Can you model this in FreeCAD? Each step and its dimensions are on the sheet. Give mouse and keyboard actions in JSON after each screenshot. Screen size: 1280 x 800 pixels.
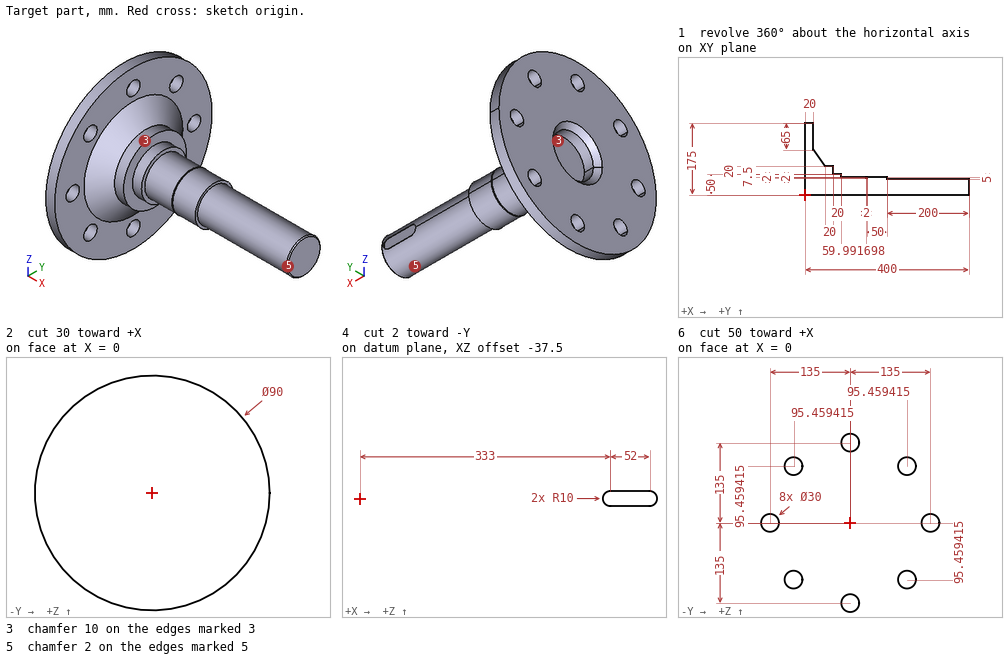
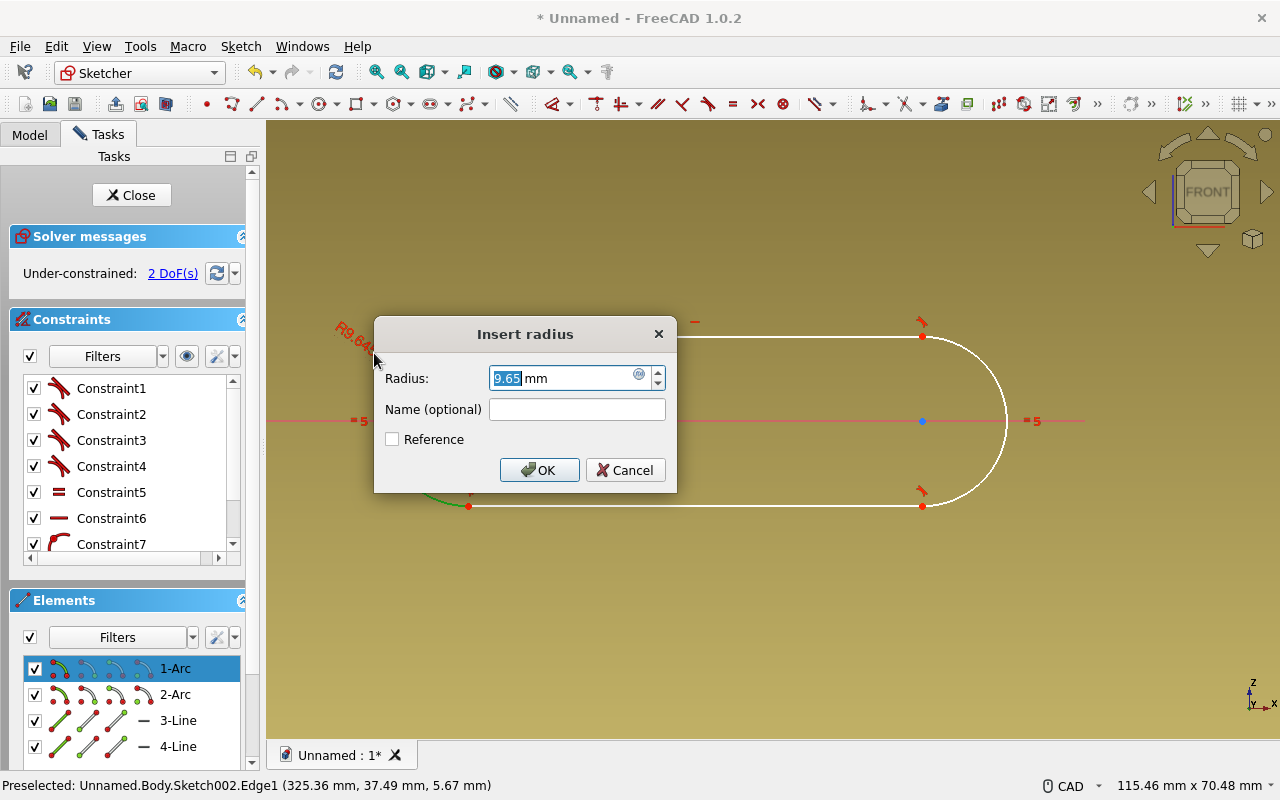
{"action": "type", "text": "10"}
{"action": "key", "text": "Return"}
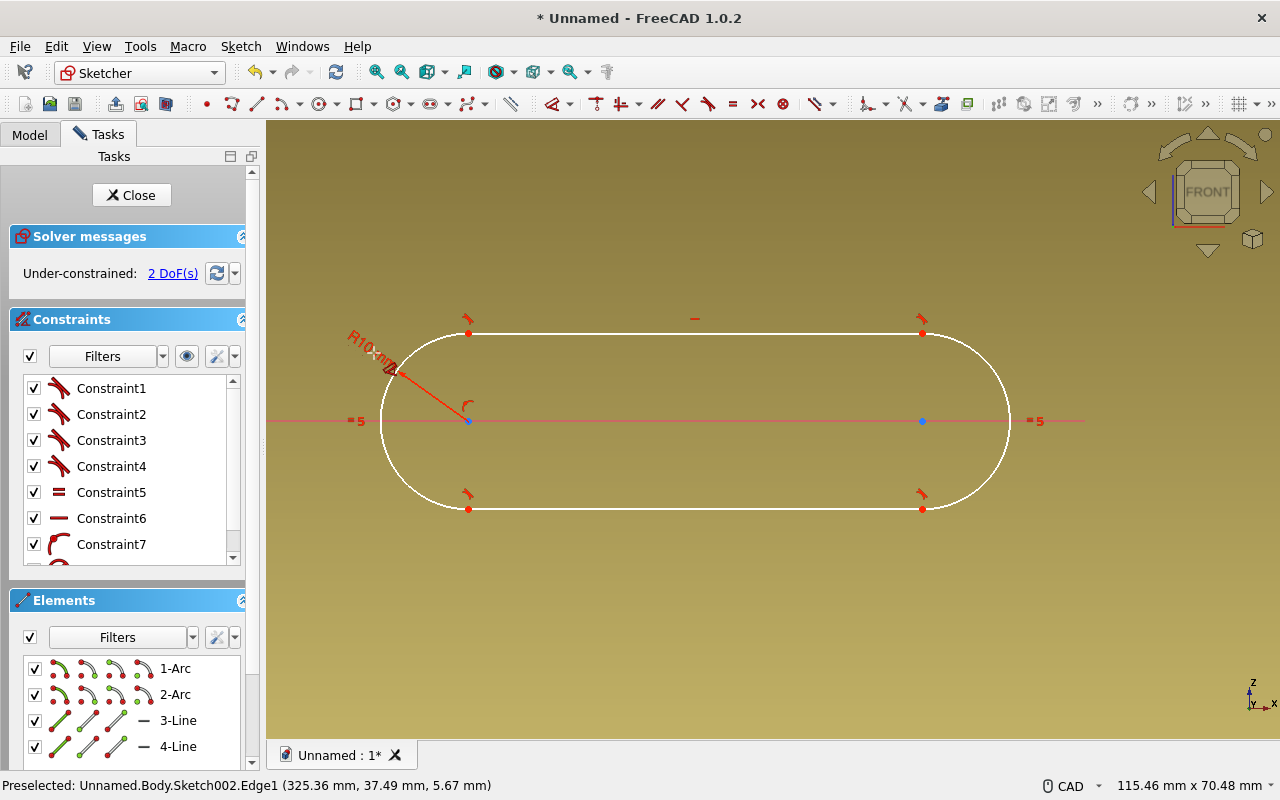
{"action": "left_click", "coordinate": [605, 334]}
{"action": "left_click", "coordinate": [695, 300]}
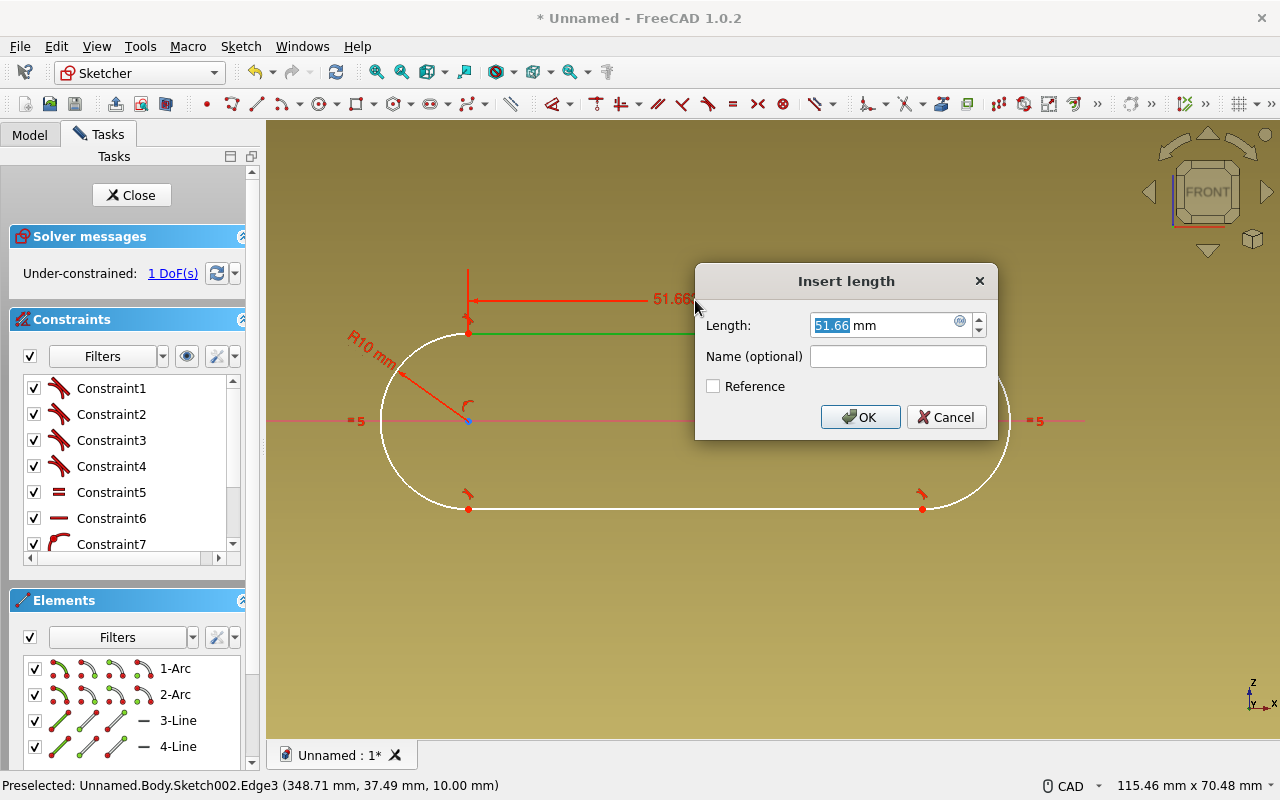
{"action": "type", "text": "52"}
{"action": "key", "text": "Return"}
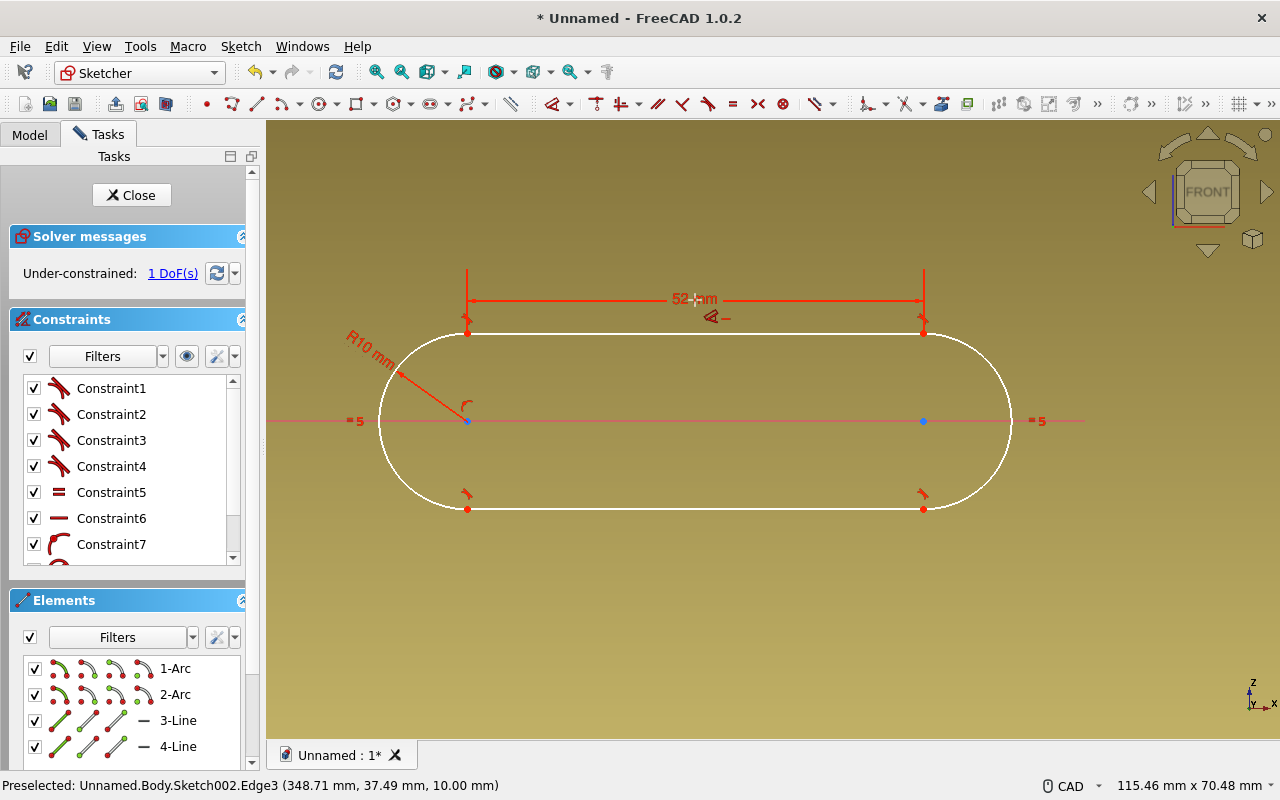
{"action": "left_click", "coordinate": [467, 334]}
{"action": "left_click", "coordinate": [381, 300]}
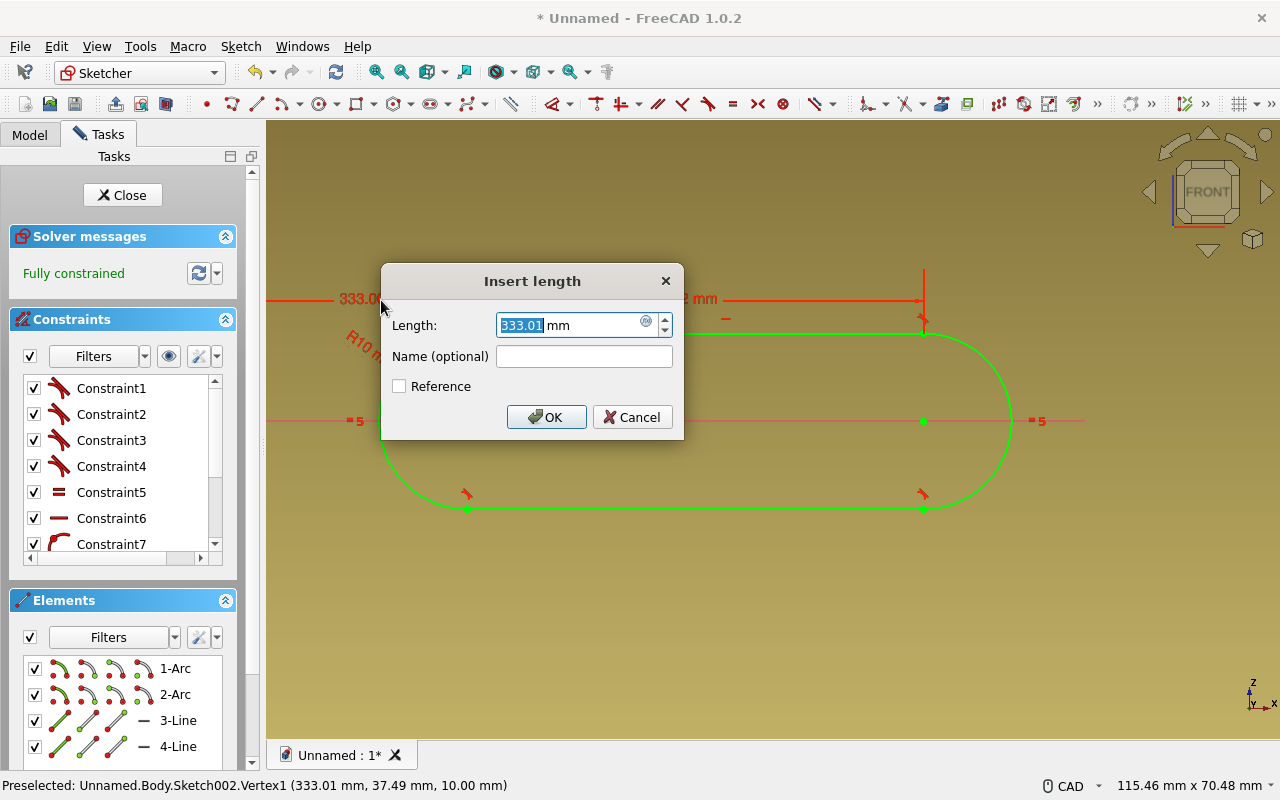
{"action": "type", "text": "333"}
{"action": "key", "text": "Return"}
{"action": "key", "text": "Escape"}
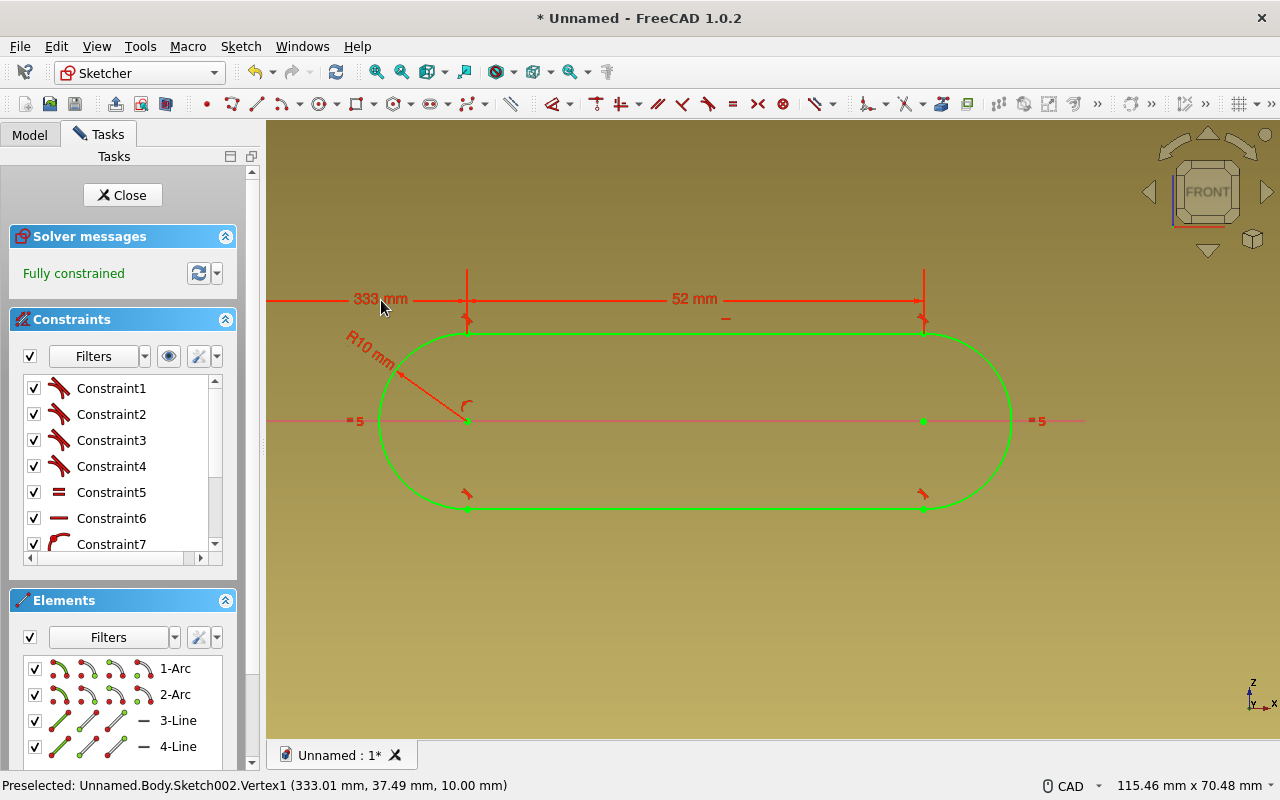
{"action": "left_click", "coordinate": [123, 195]}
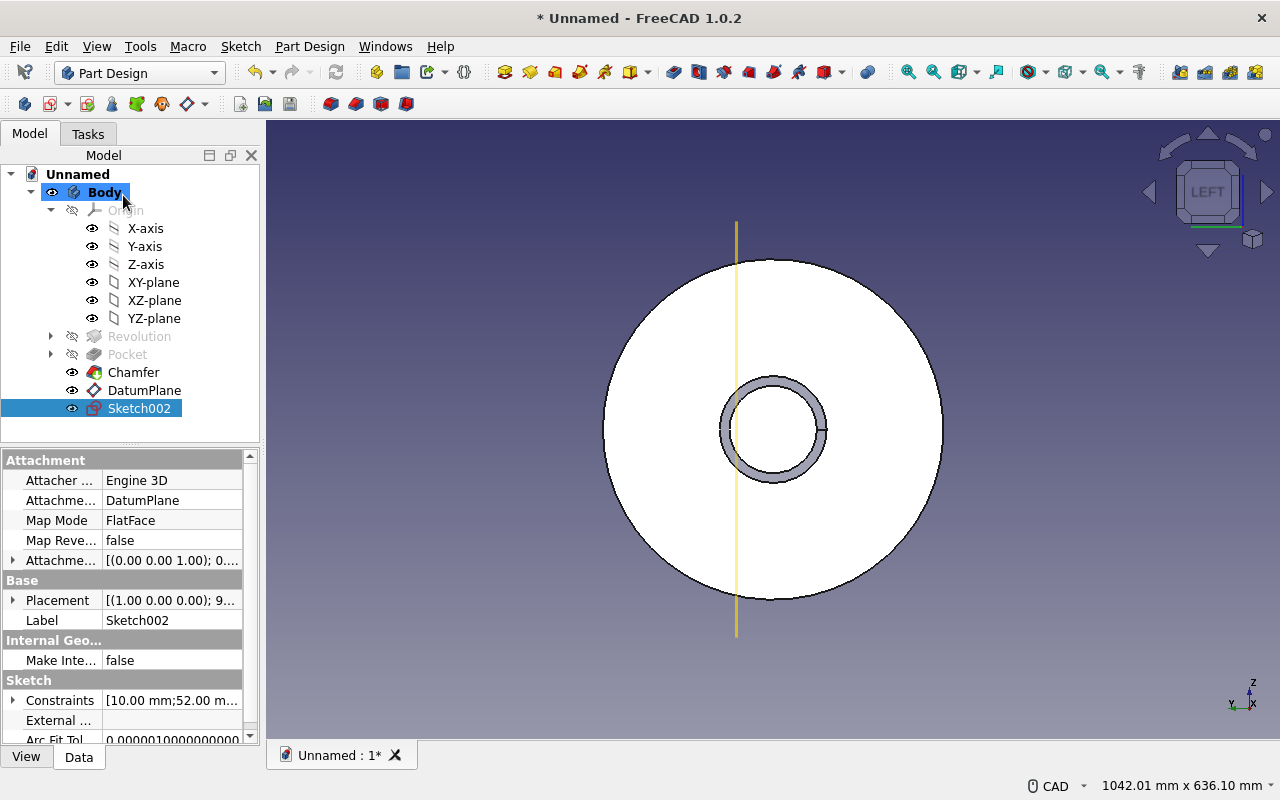
{"action": "left_click", "coordinate": [674, 72]}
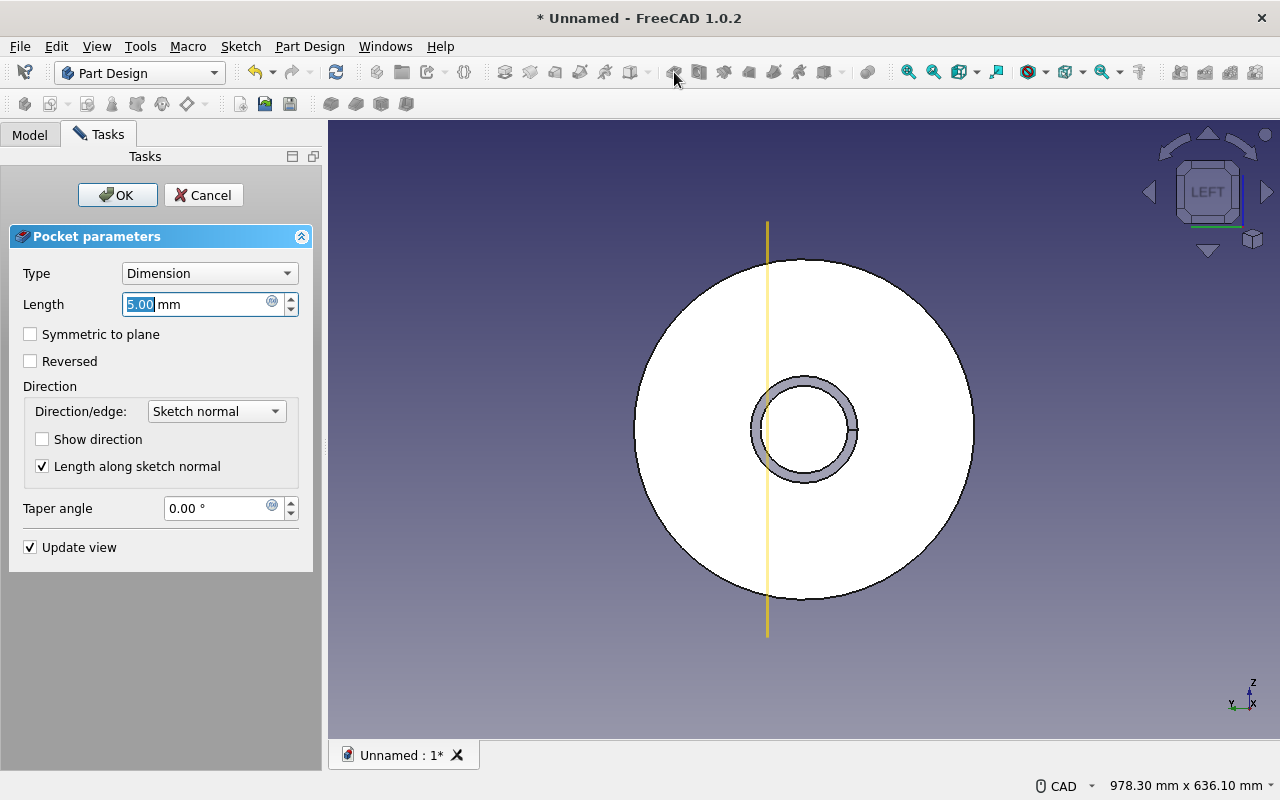
{"action": "type", "text": "2"}
{"action": "key", "text": "Tab"}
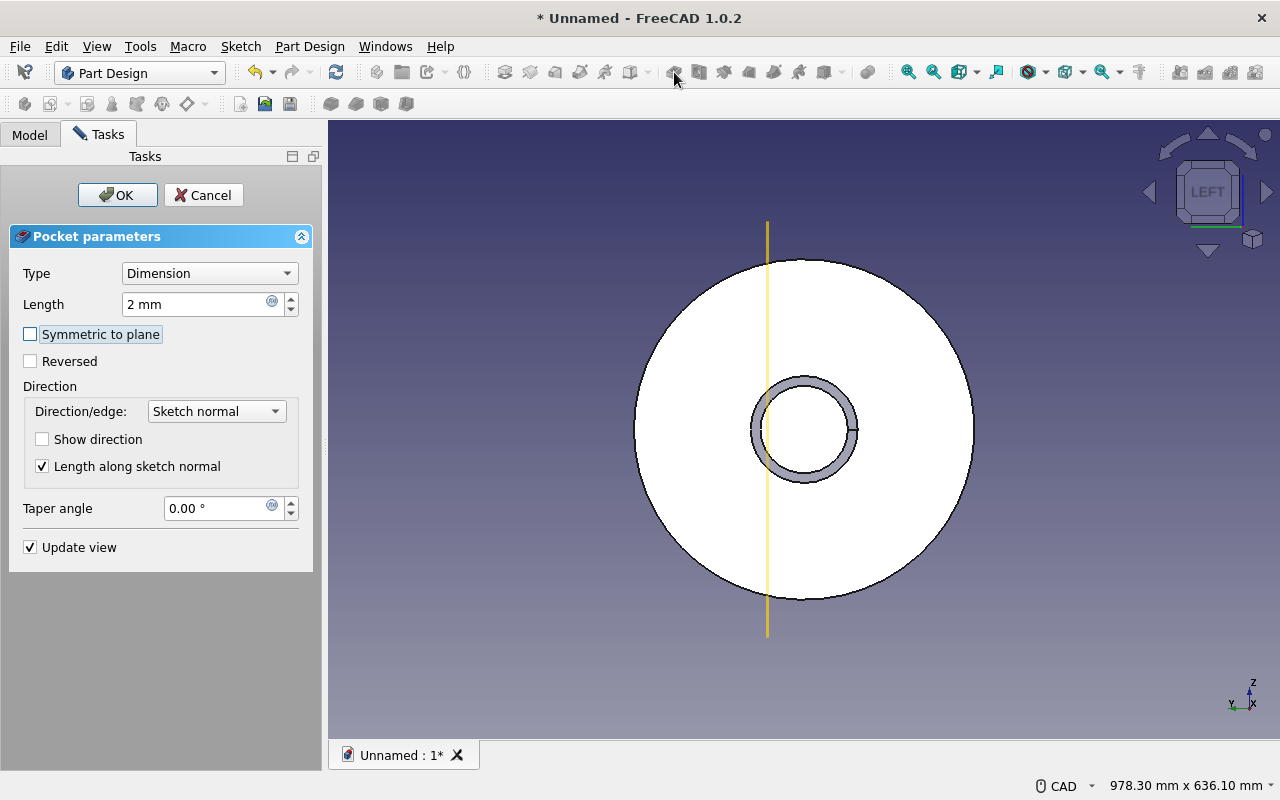
{"action": "left_click", "coordinate": [31, 361]}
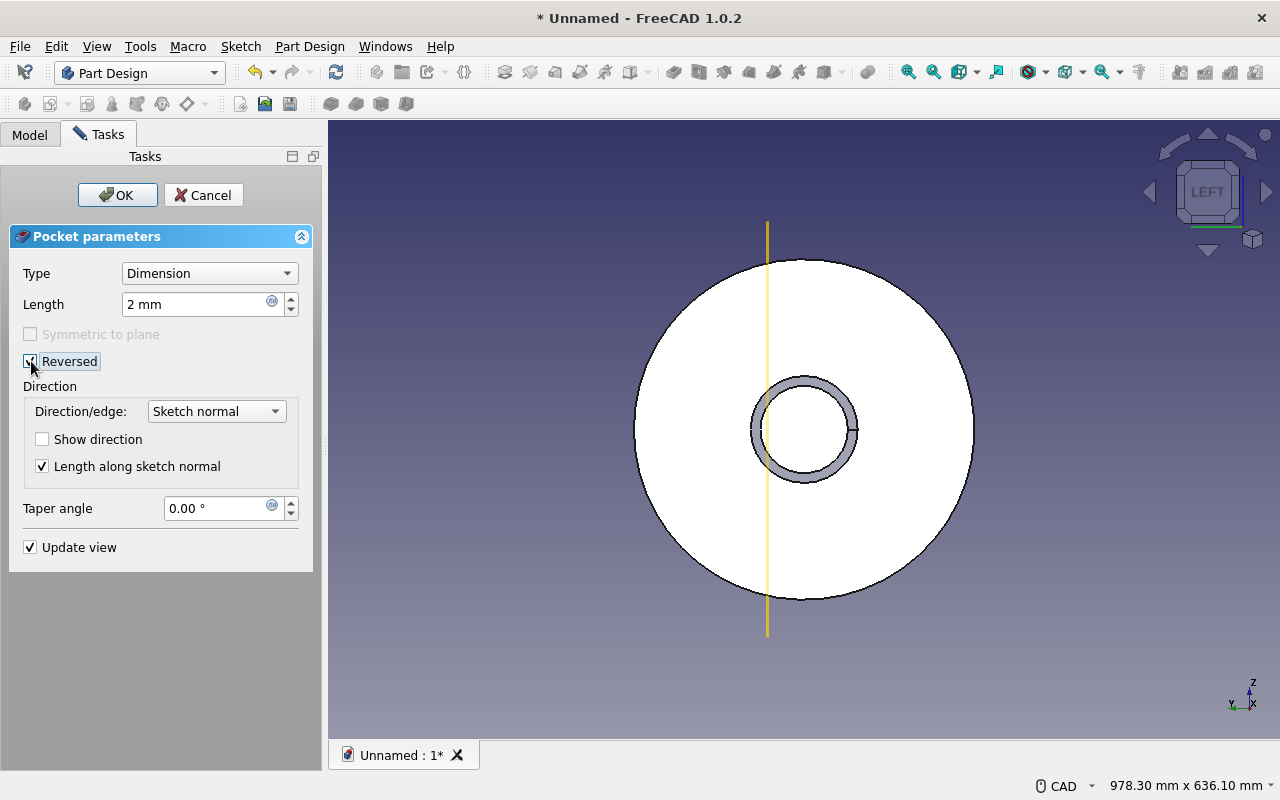
{"action": "left_click", "coordinate": [118, 195]}